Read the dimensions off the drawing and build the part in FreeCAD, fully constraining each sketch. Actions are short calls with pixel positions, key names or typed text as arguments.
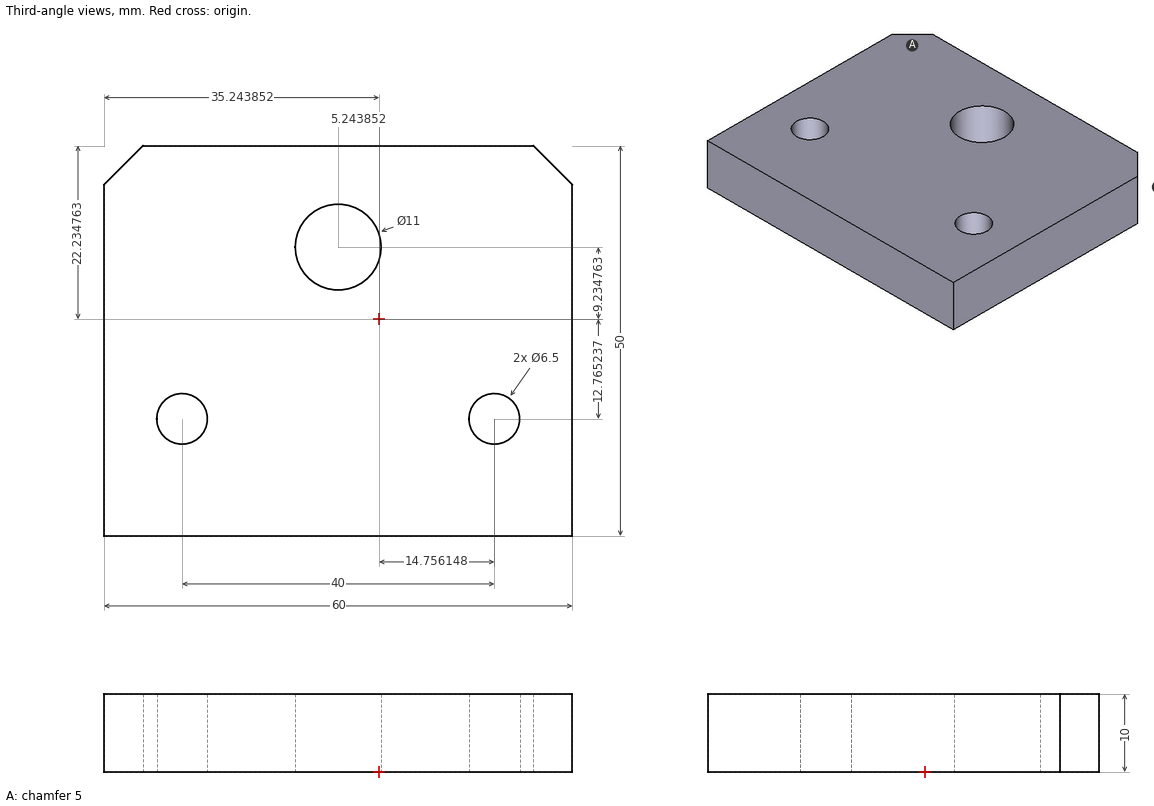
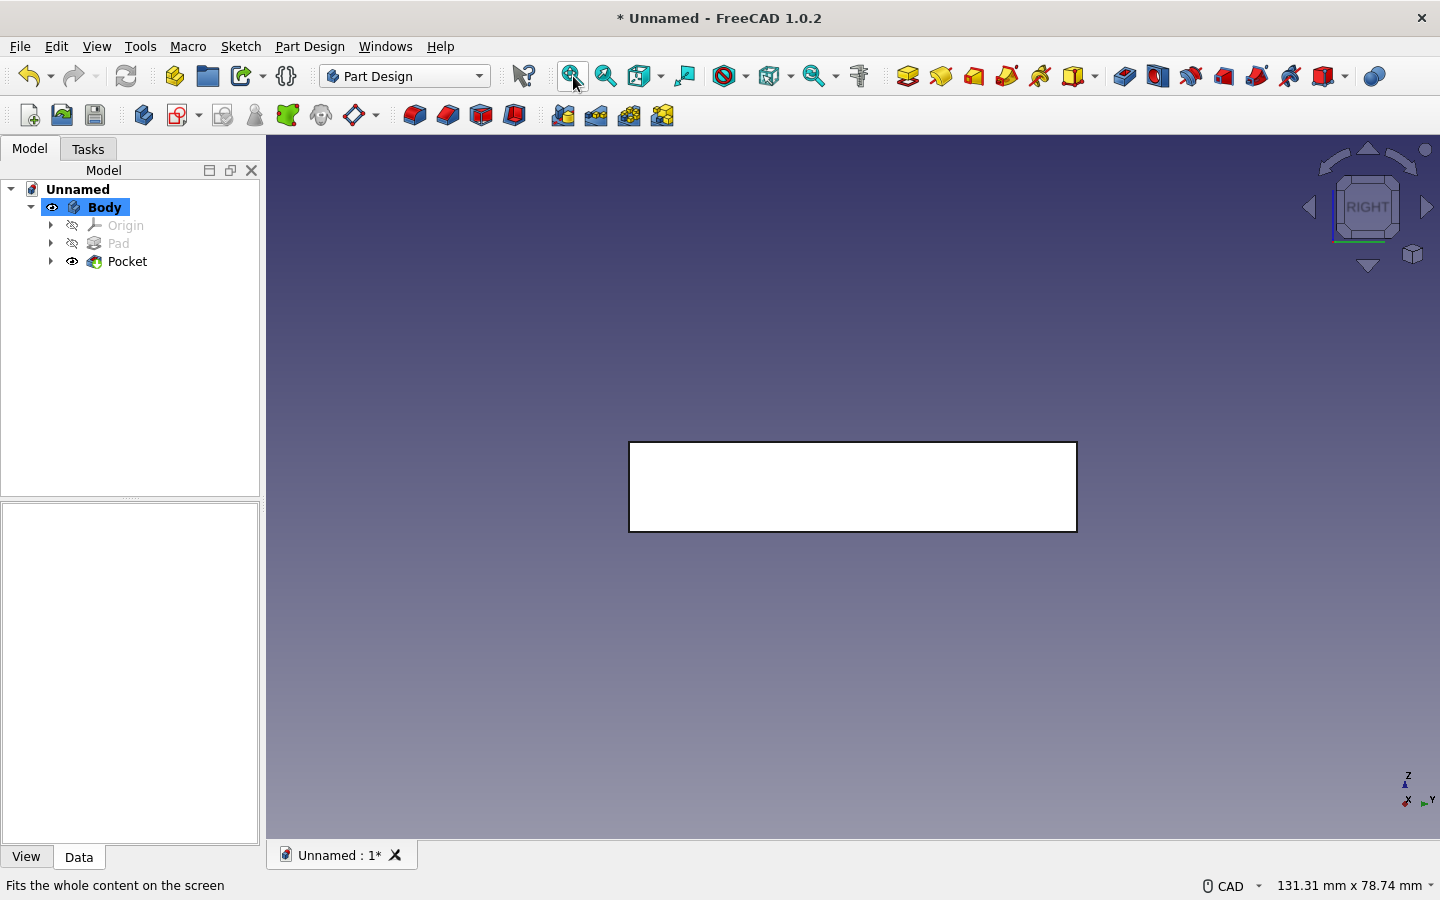
click(1077, 486)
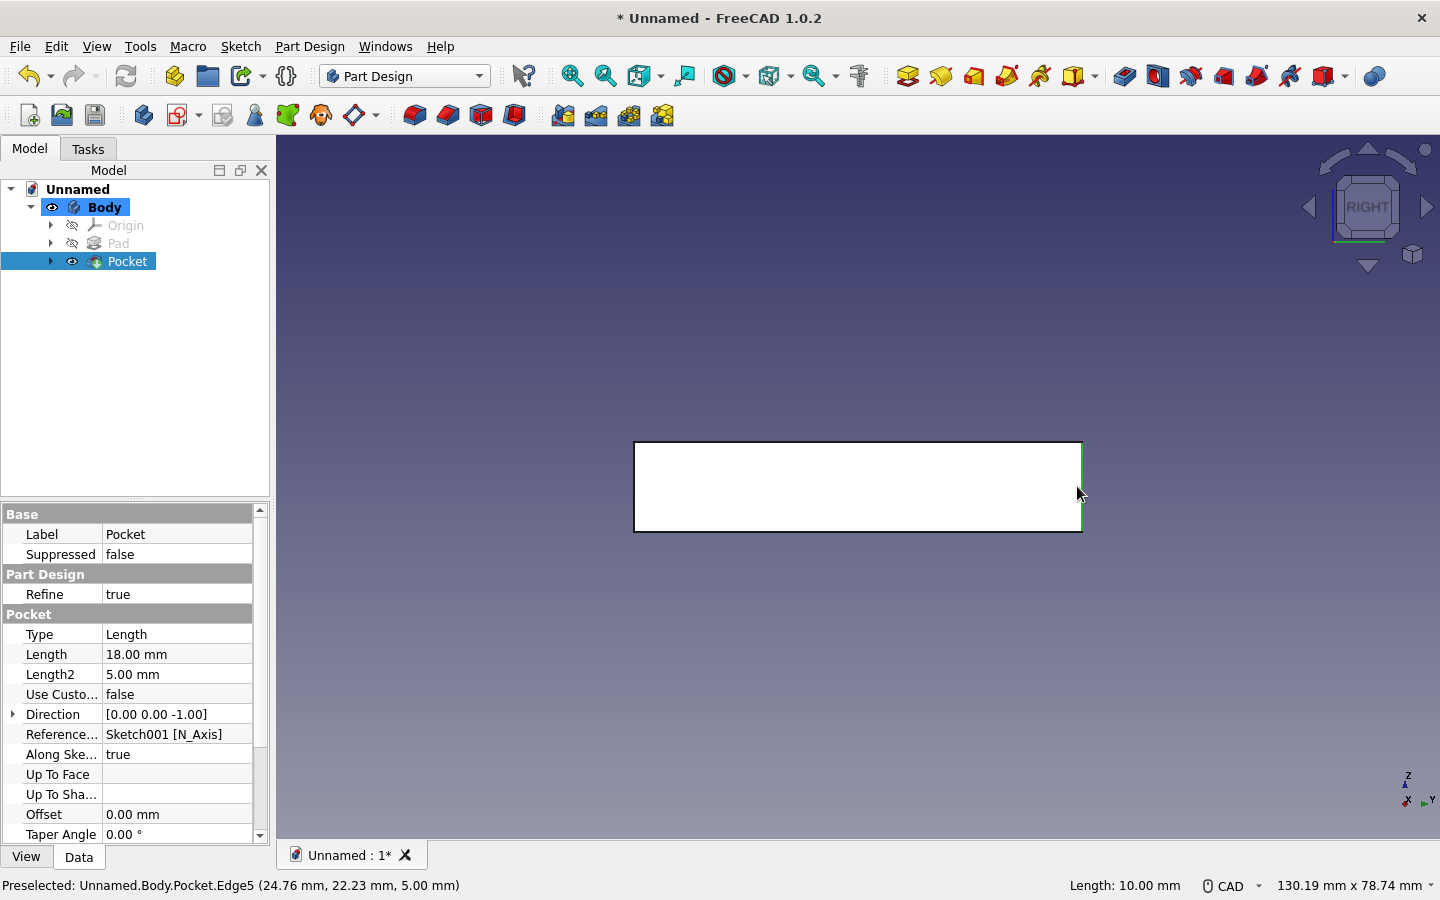
key(5)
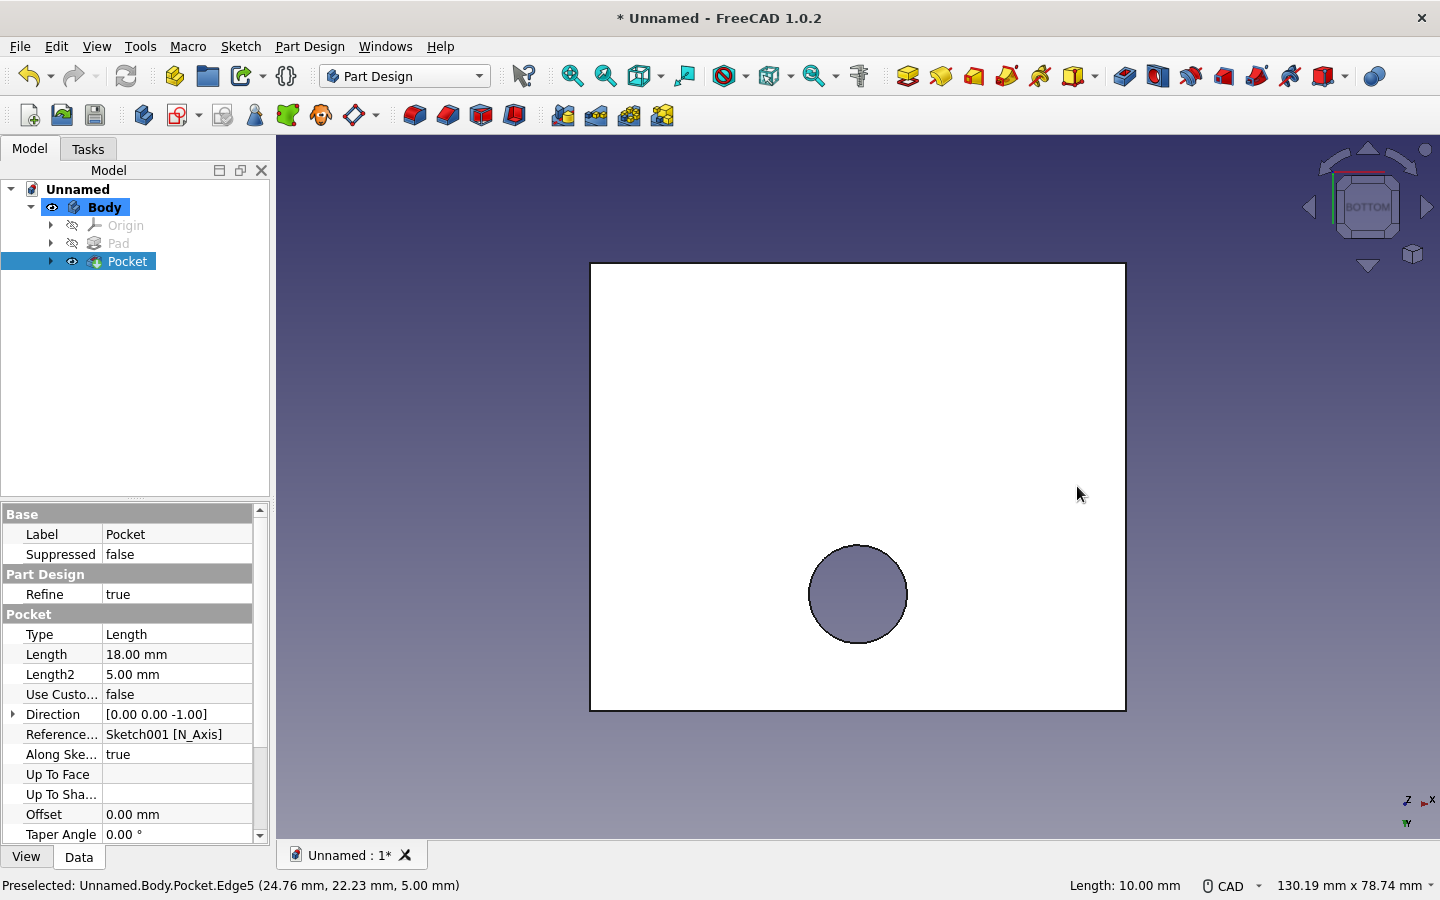
key(4)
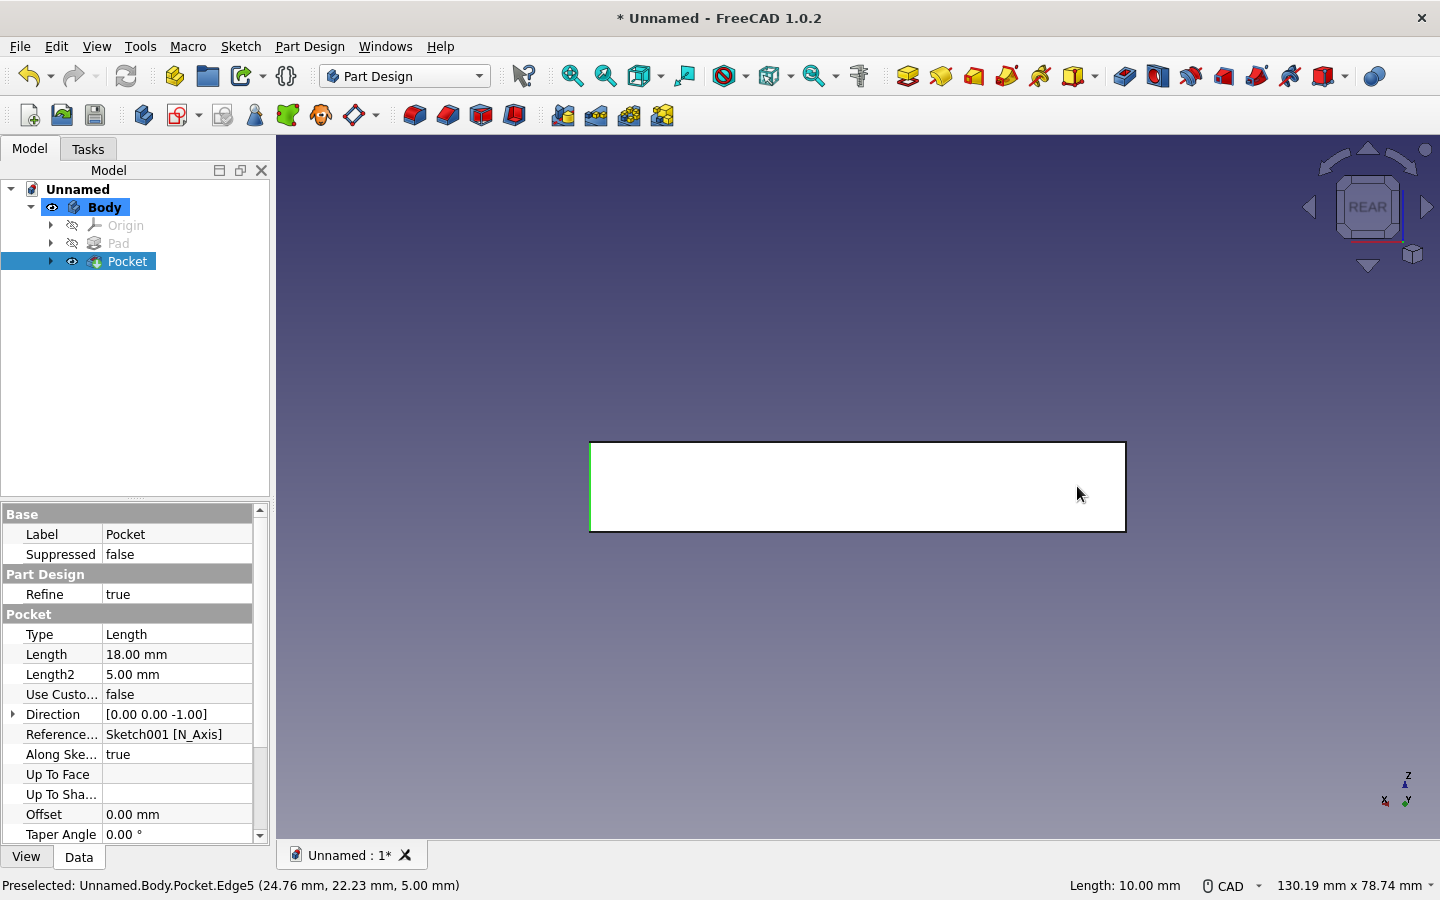
click(1126, 486, ctrl)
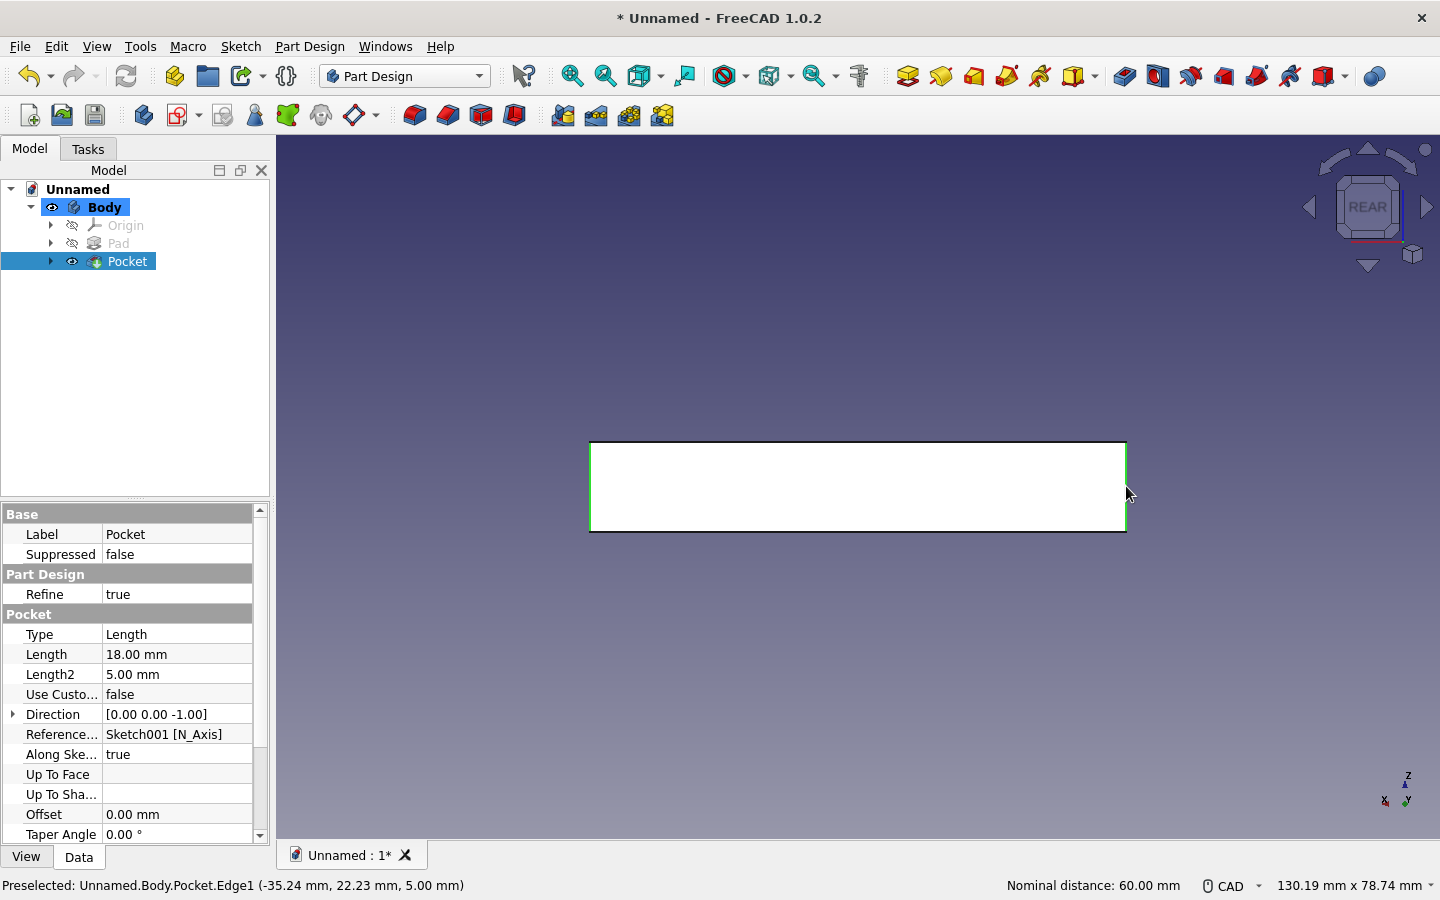
click(448, 116)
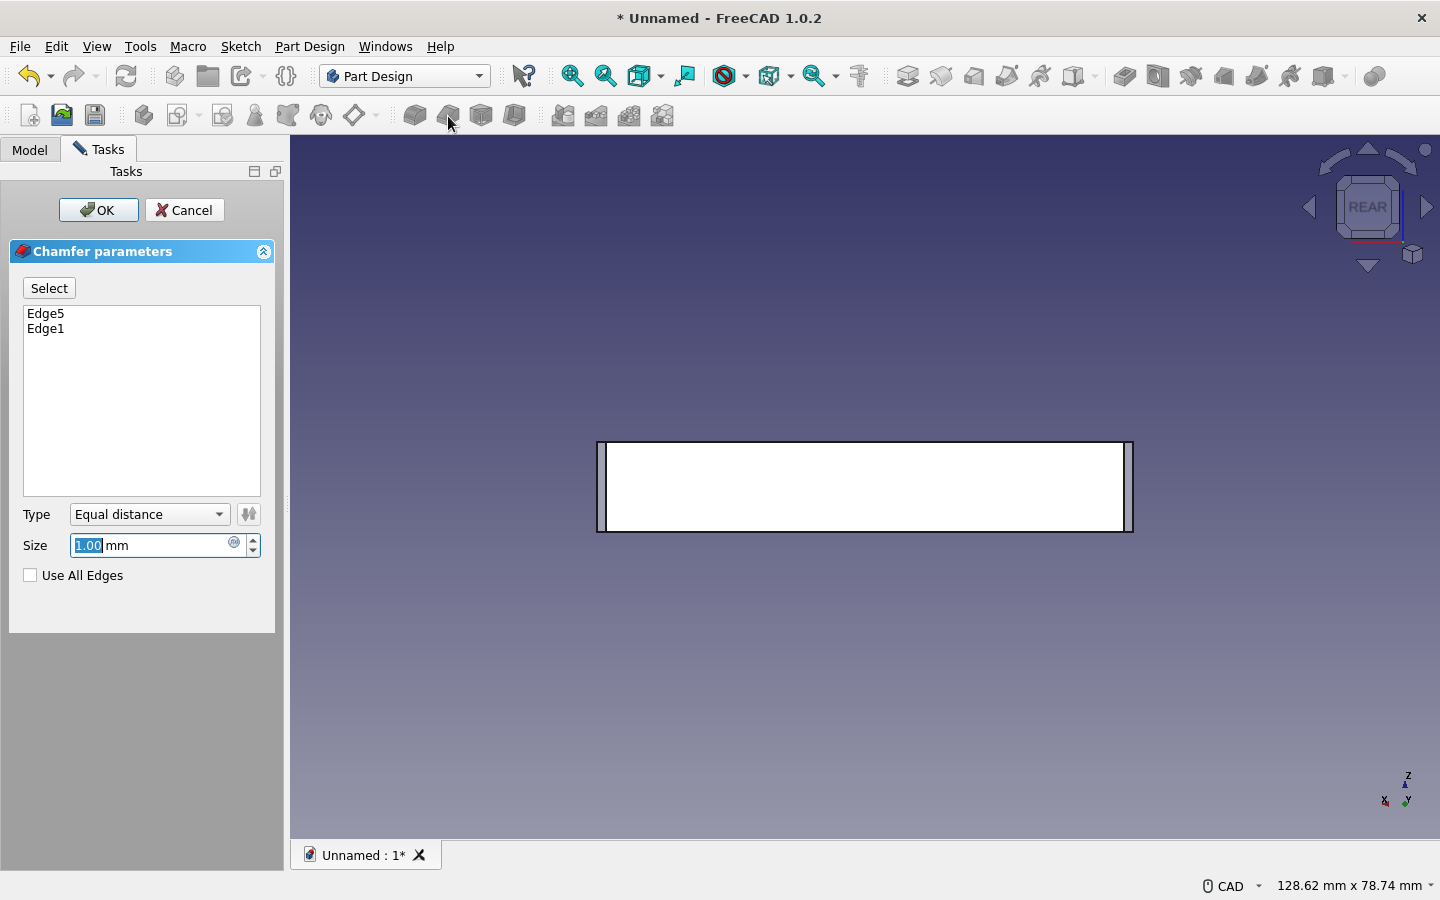
text(5)
key(Tab)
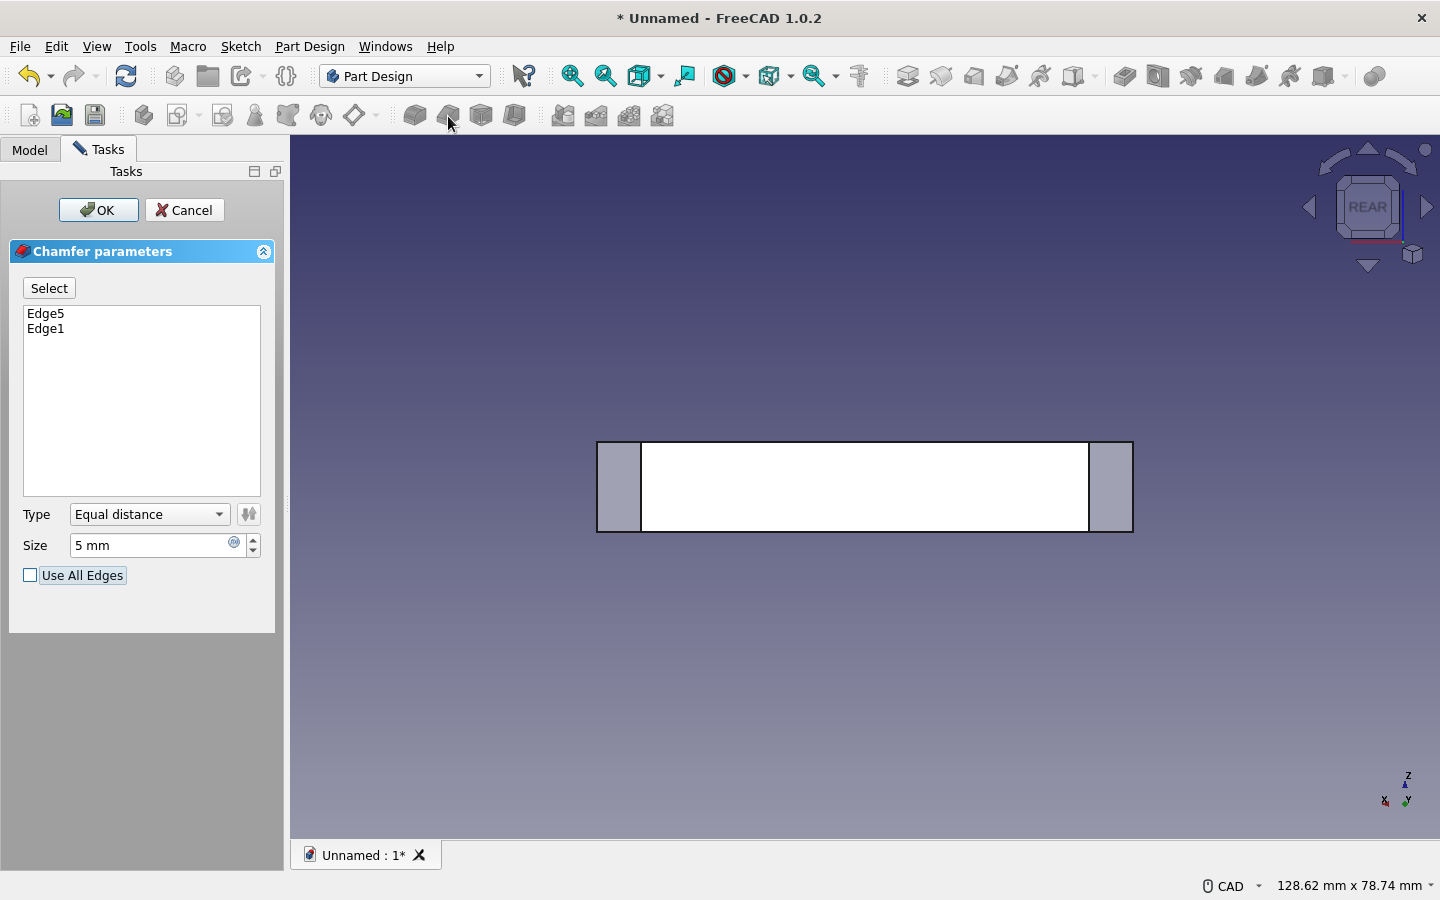
click(99, 210)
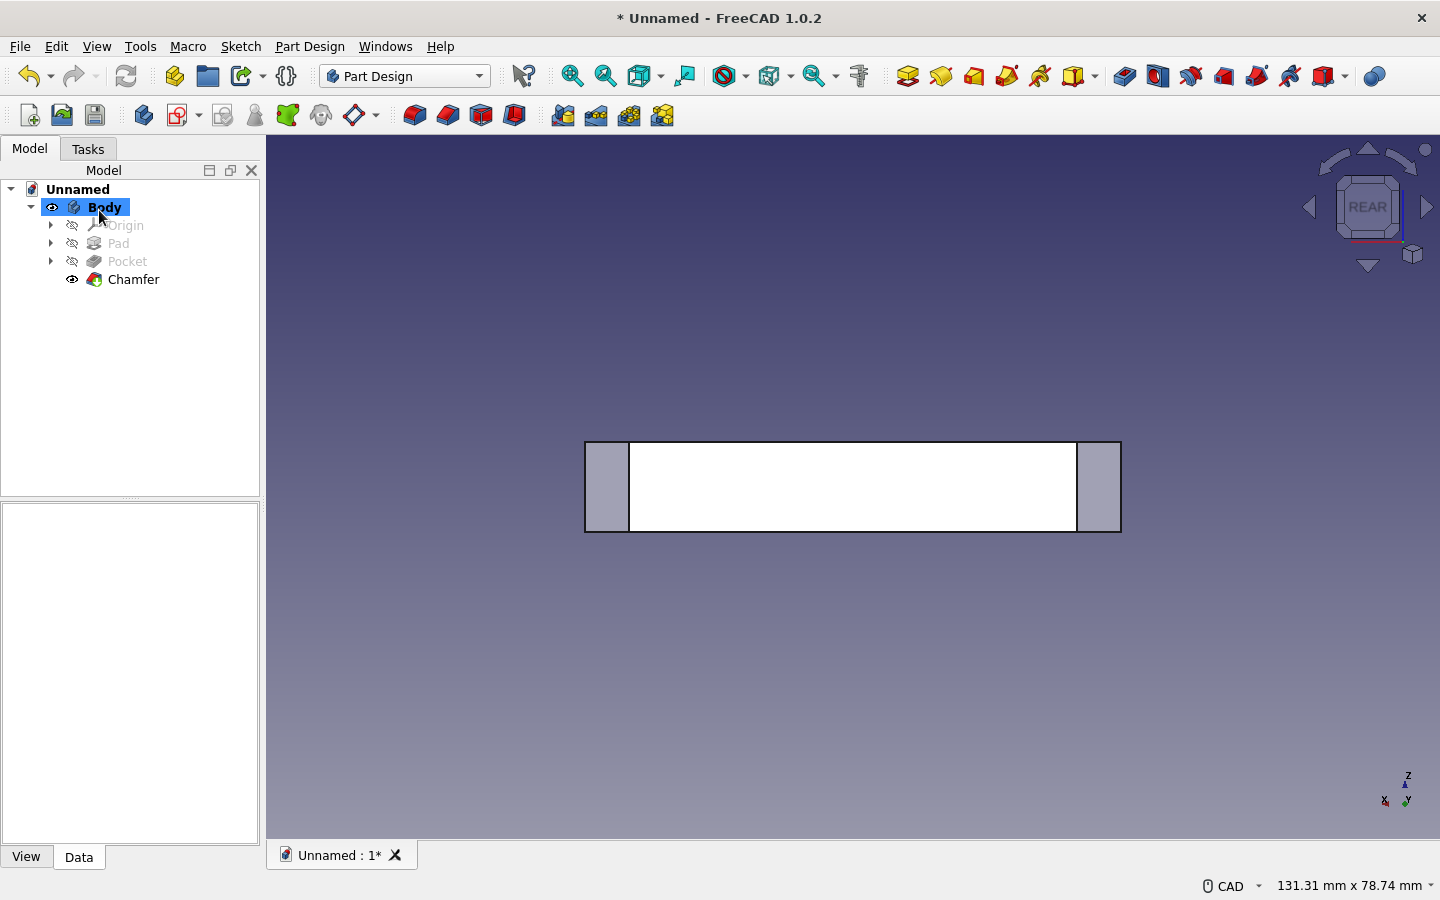
key(5)